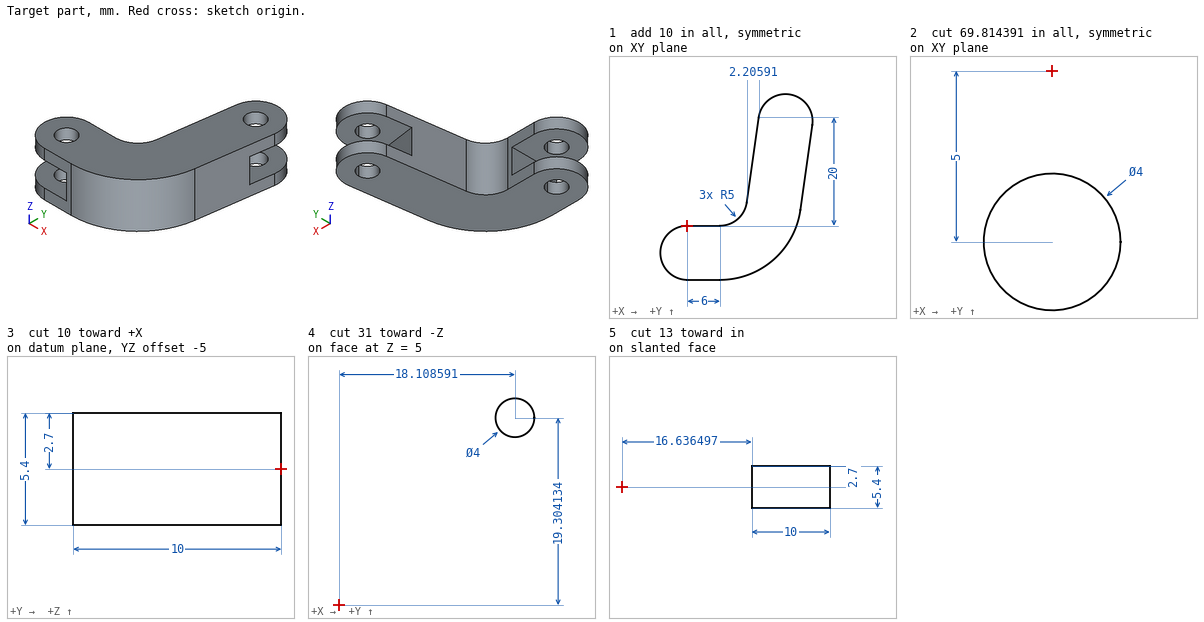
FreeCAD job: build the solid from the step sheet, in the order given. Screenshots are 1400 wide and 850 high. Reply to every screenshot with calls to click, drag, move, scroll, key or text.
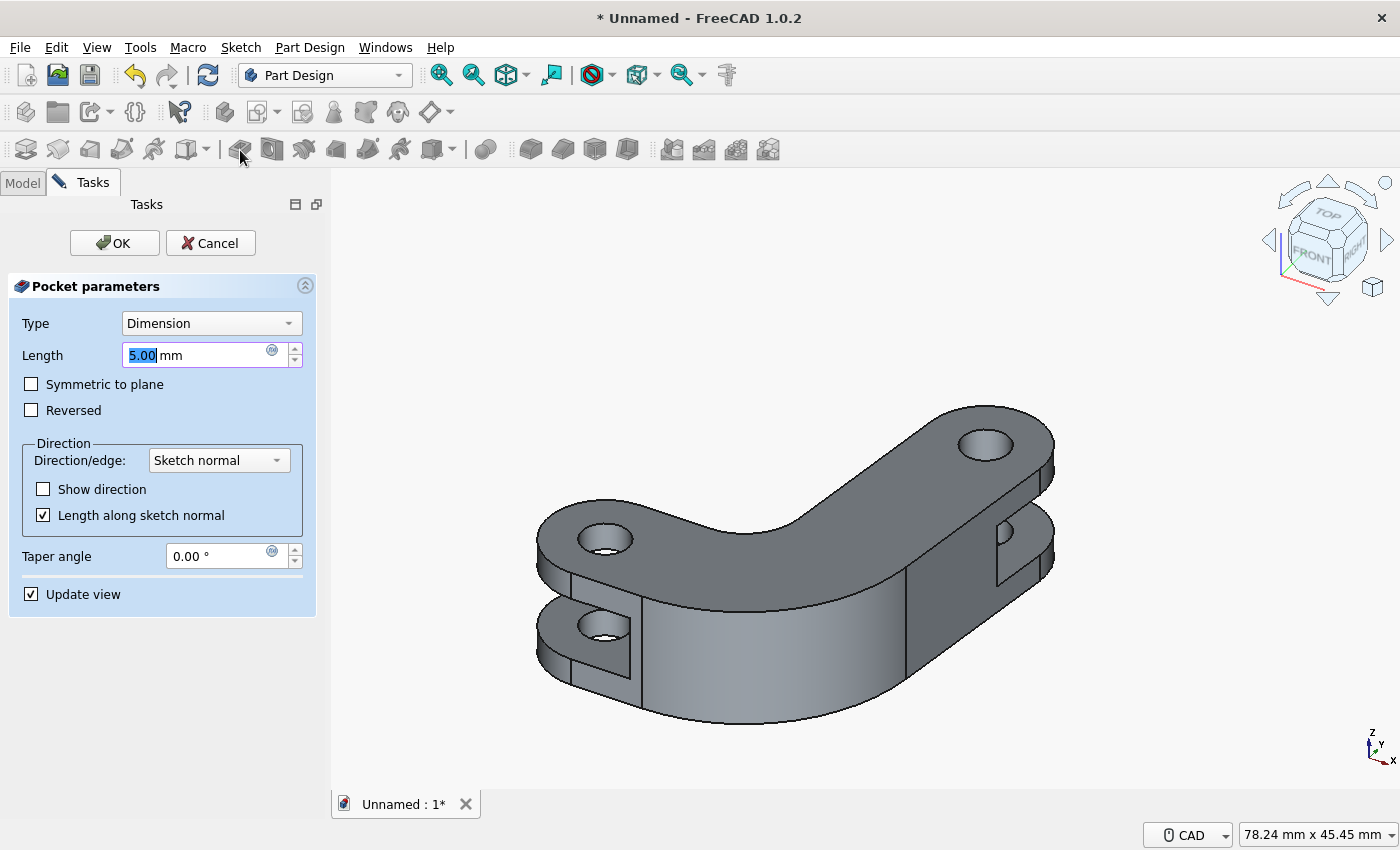
text(13)
key(Tab)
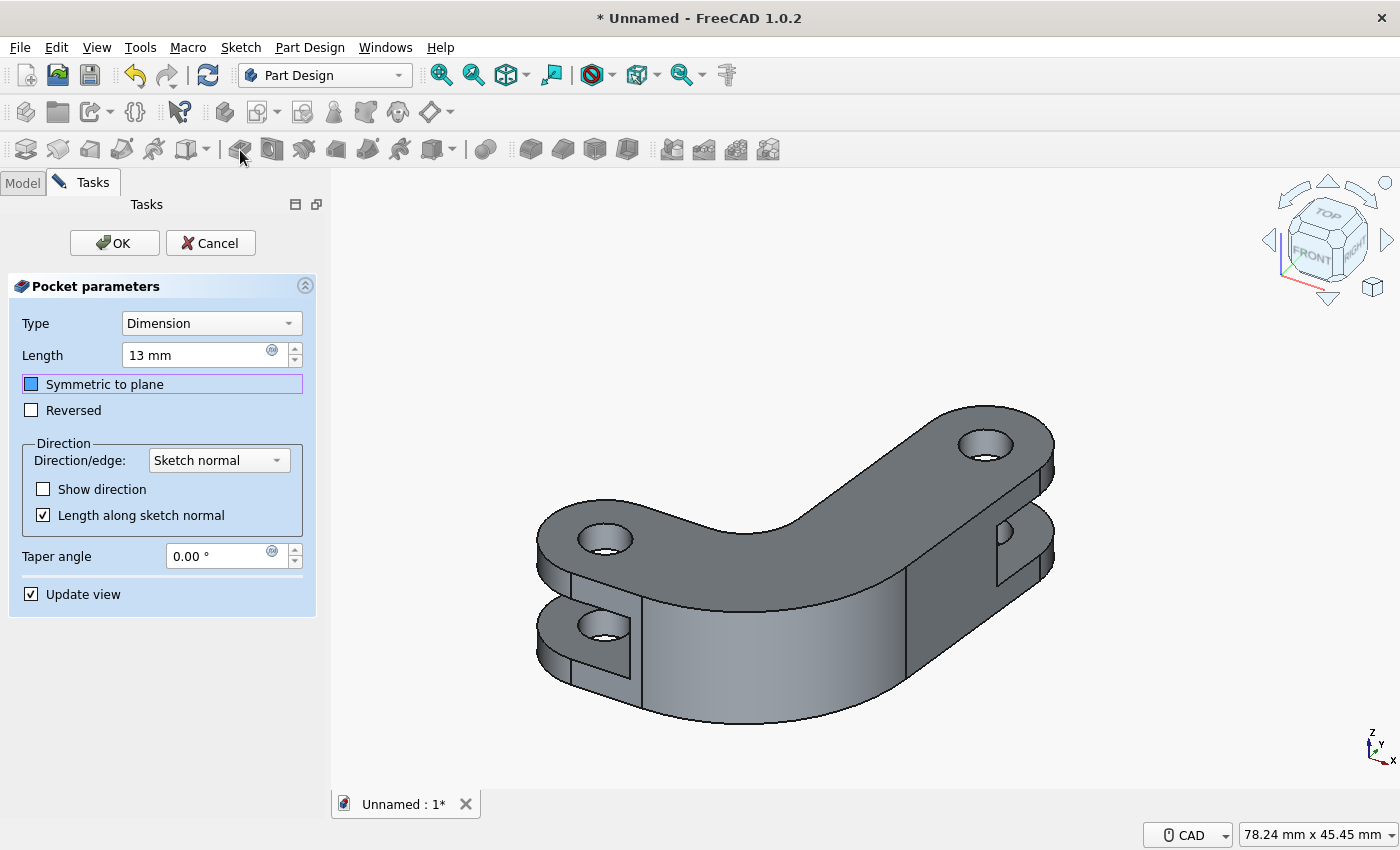
click(115, 243)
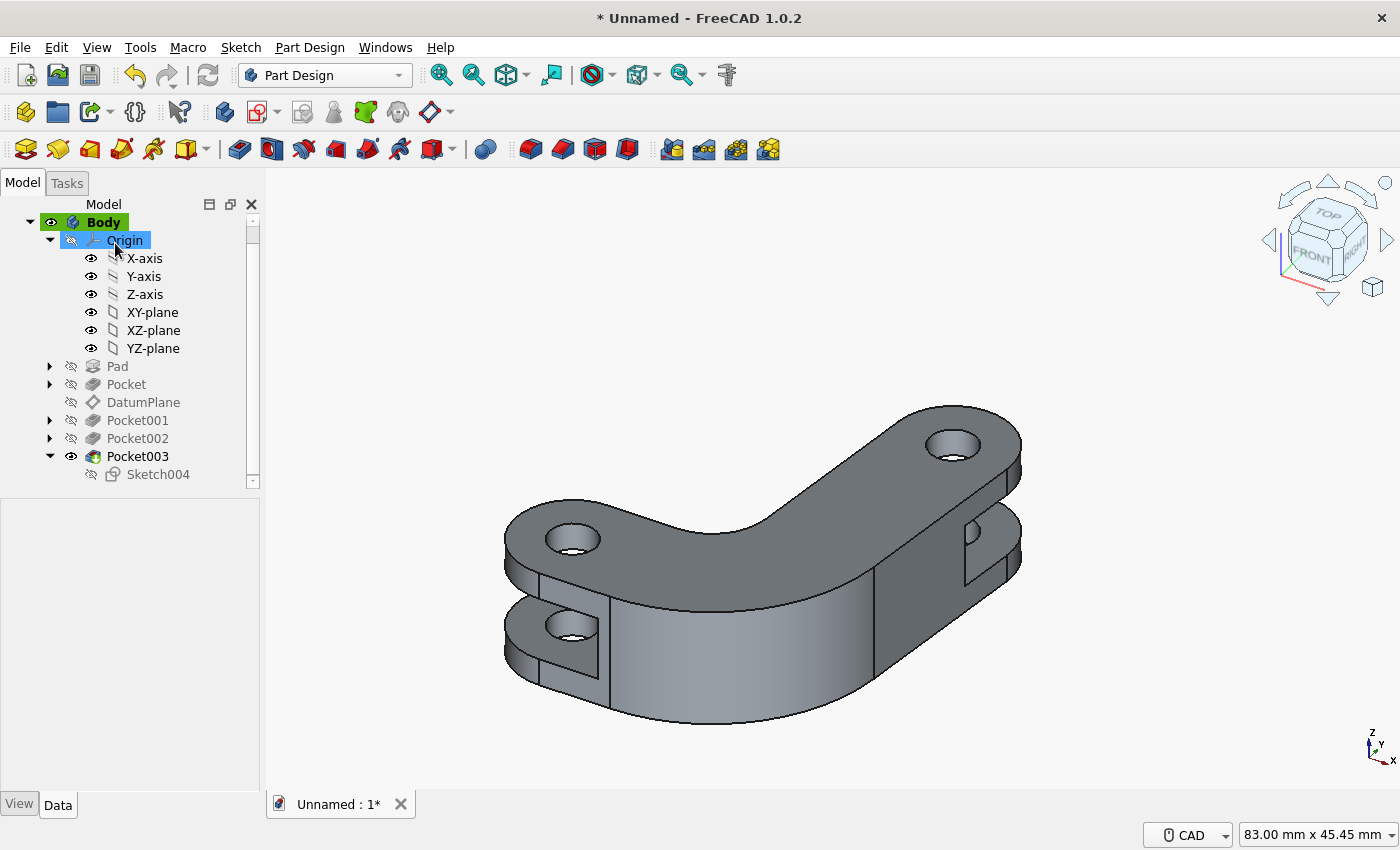
key(0)